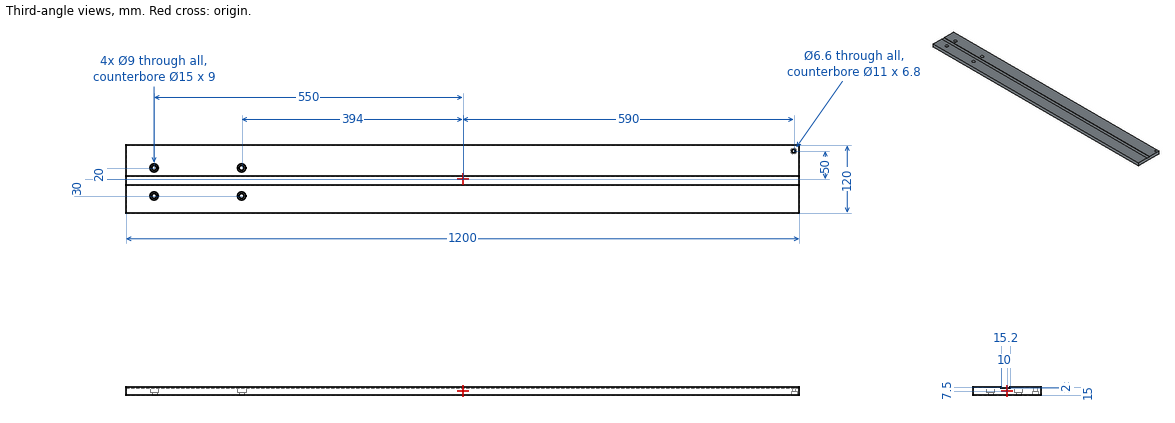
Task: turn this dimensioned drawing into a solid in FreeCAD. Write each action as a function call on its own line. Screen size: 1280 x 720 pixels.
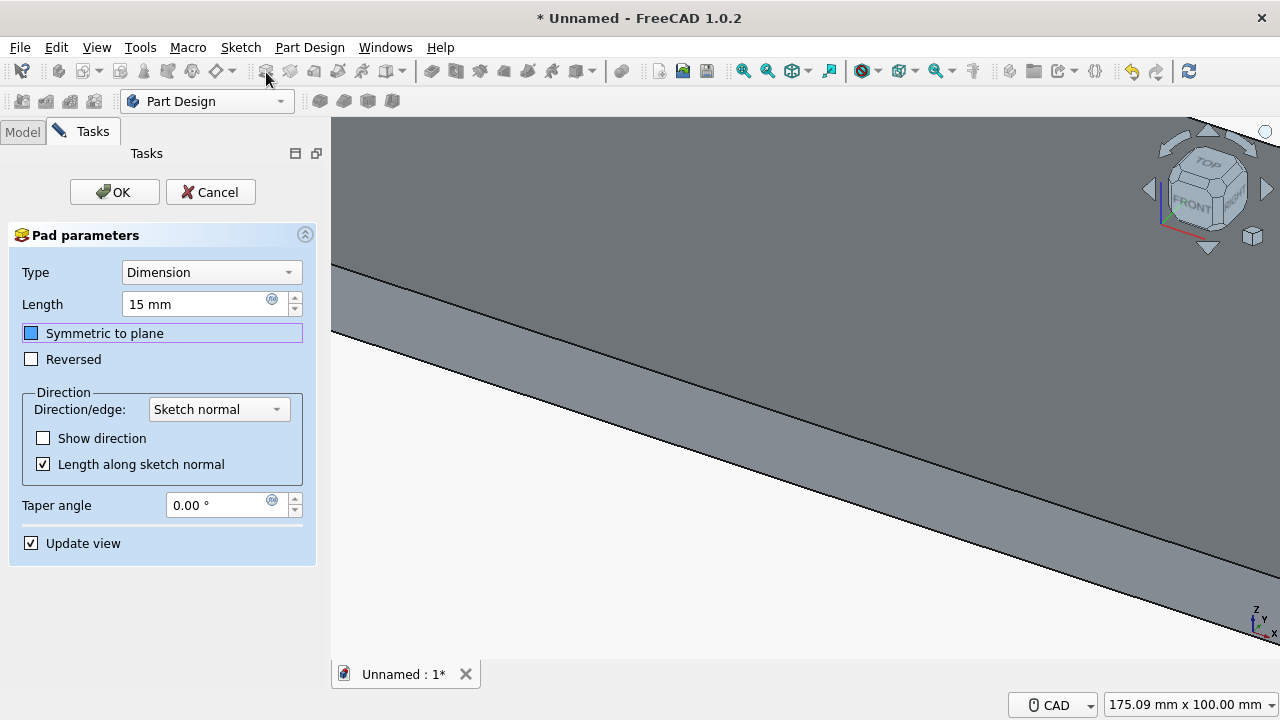
click(30, 333)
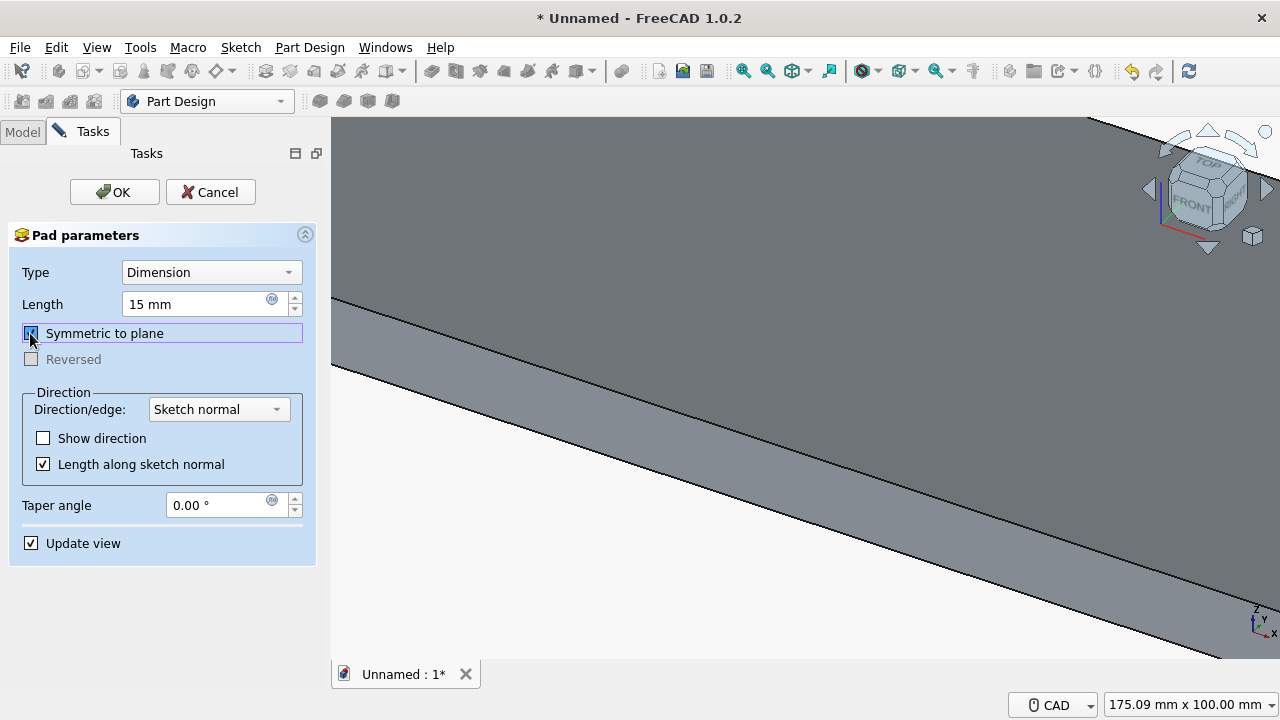
click(115, 192)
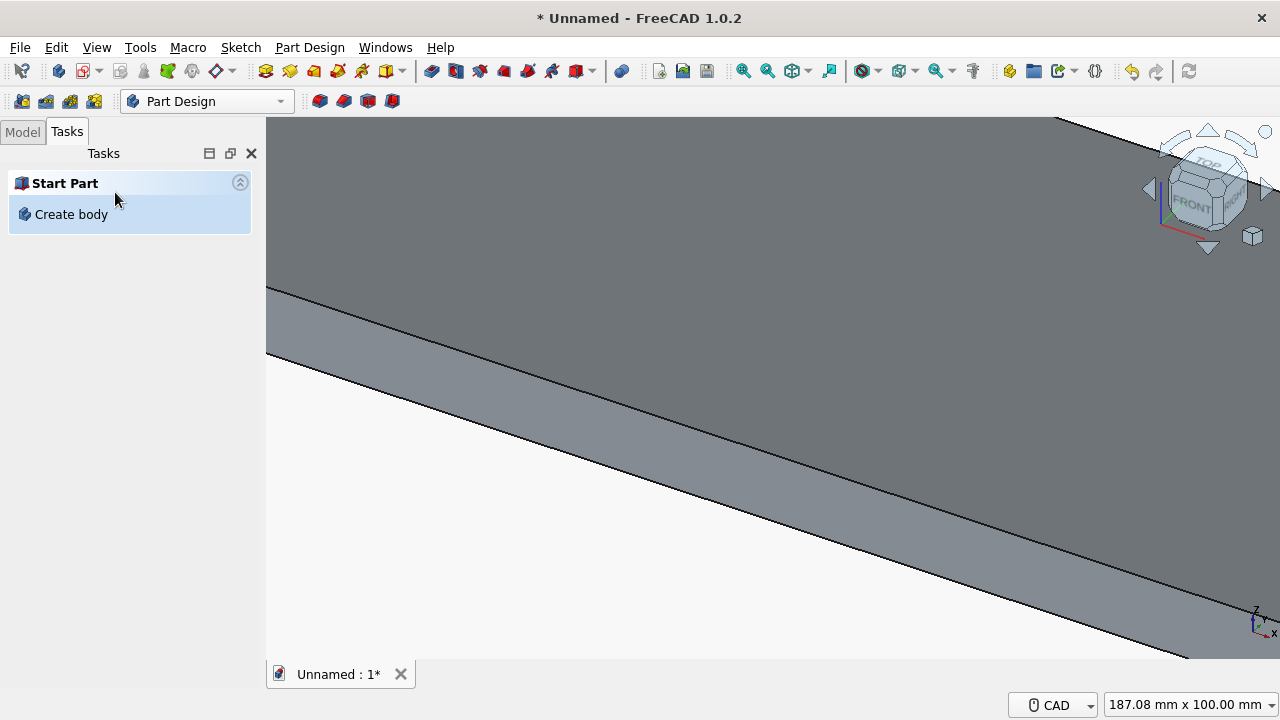
click(744, 72)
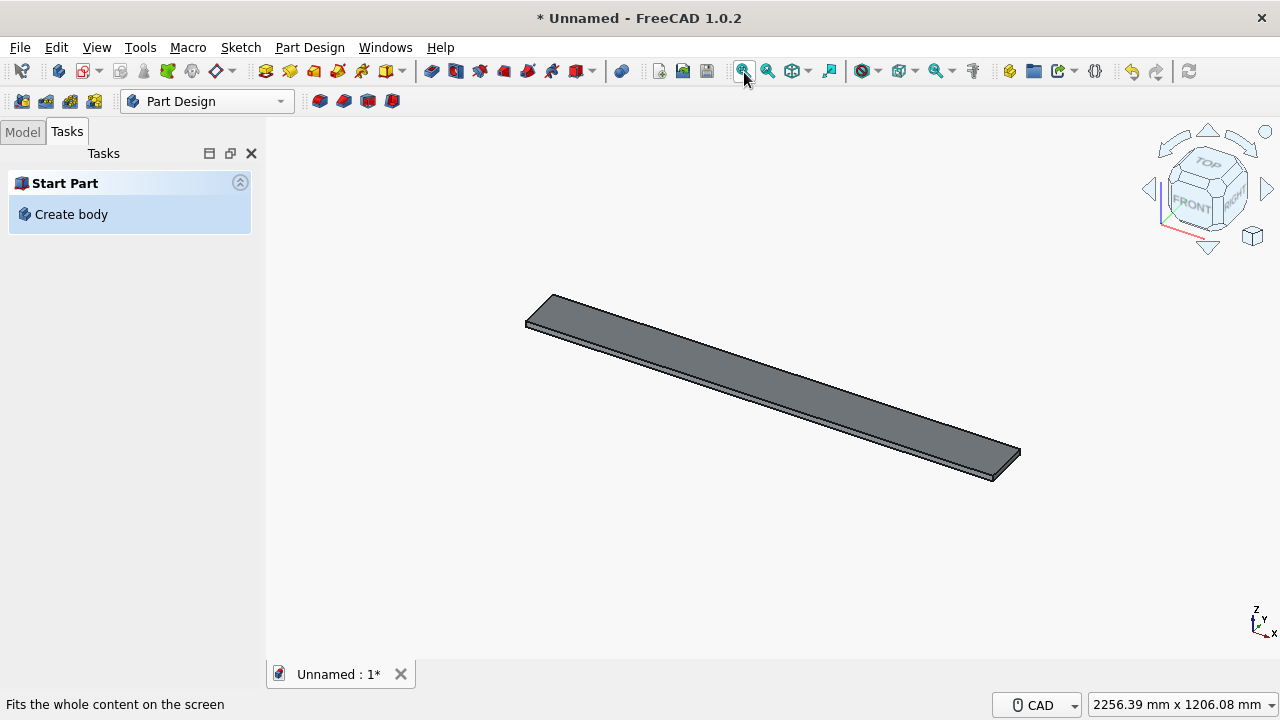
key(5)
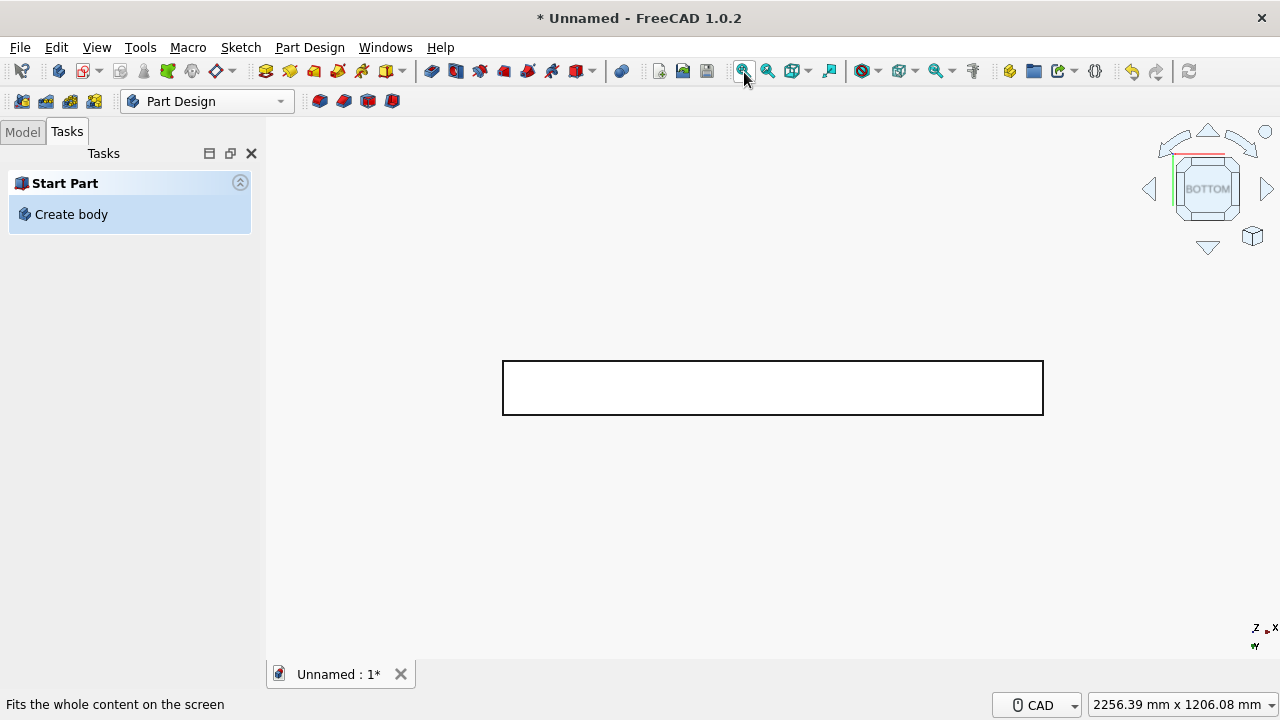
click(1004, 387)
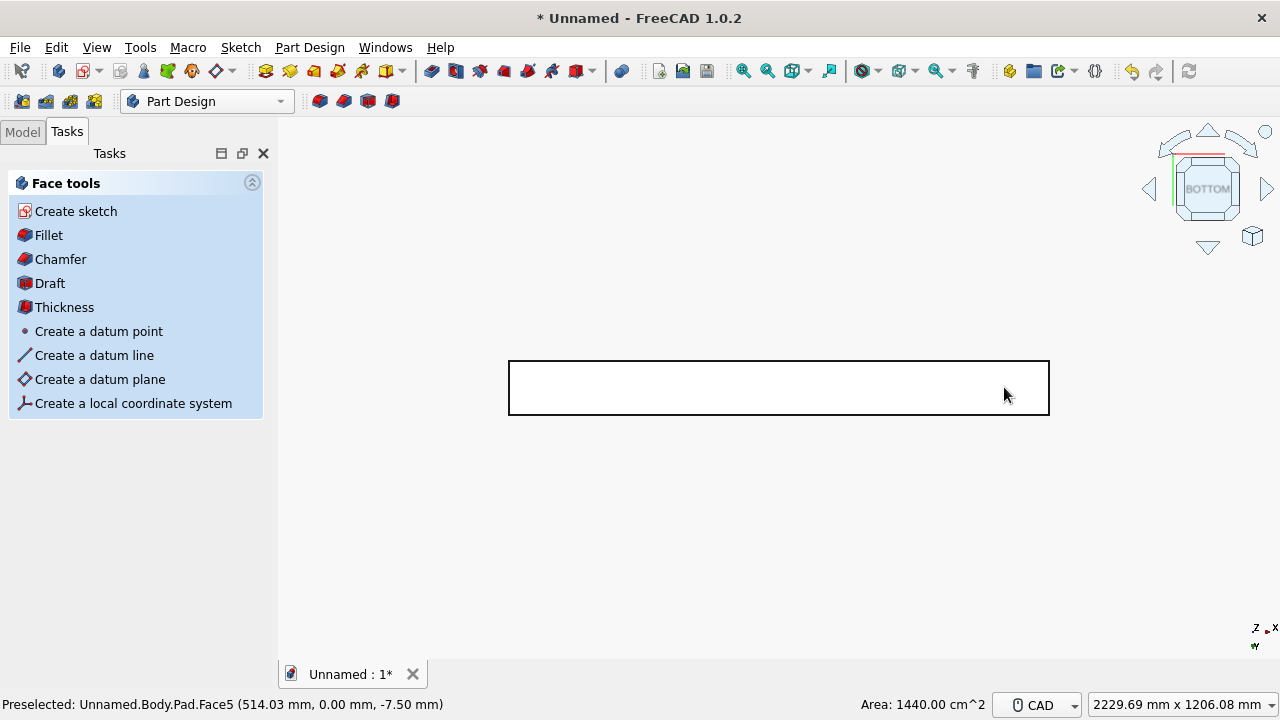
click(84, 72)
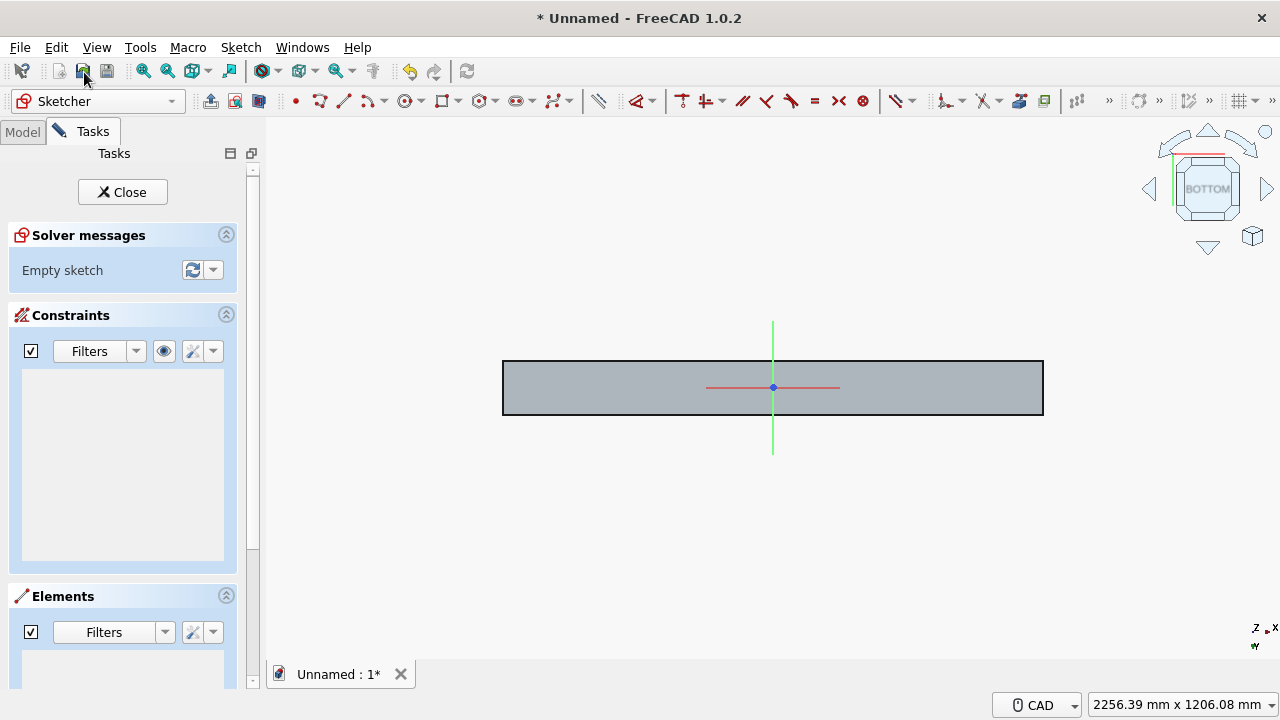
scroll(1056, 412, up, 15)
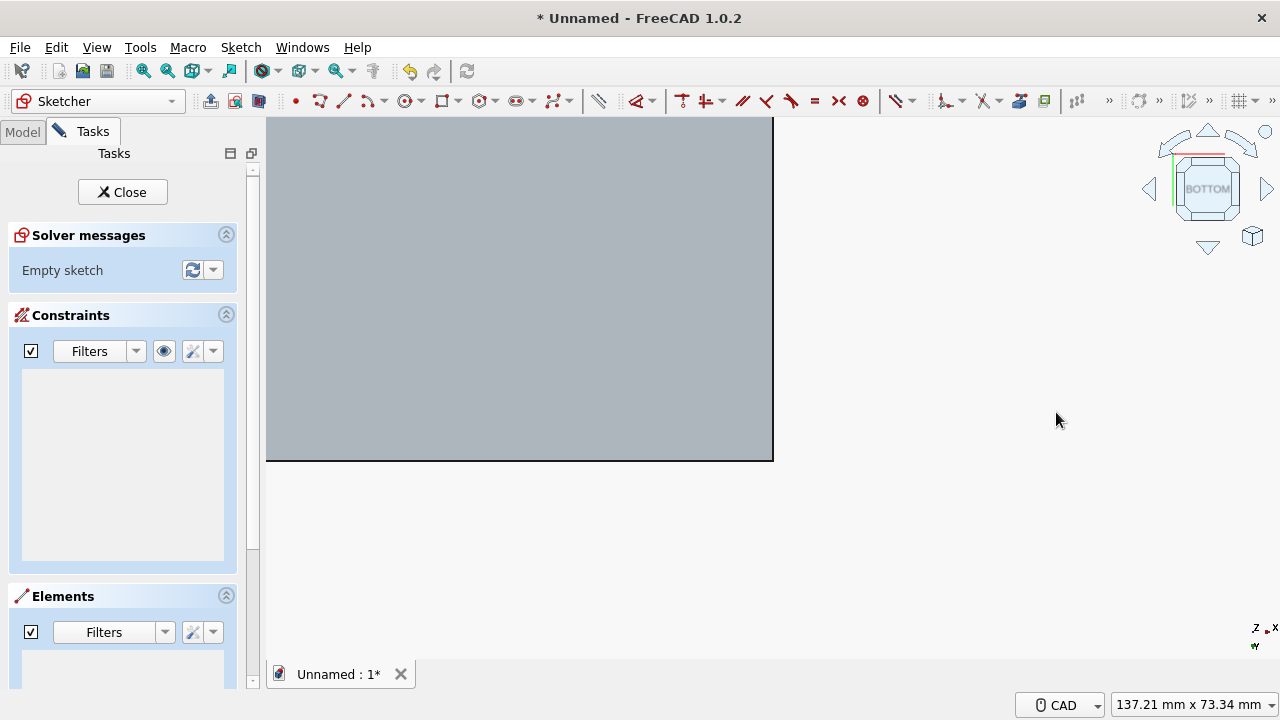
scroll(678, 367, up, 9)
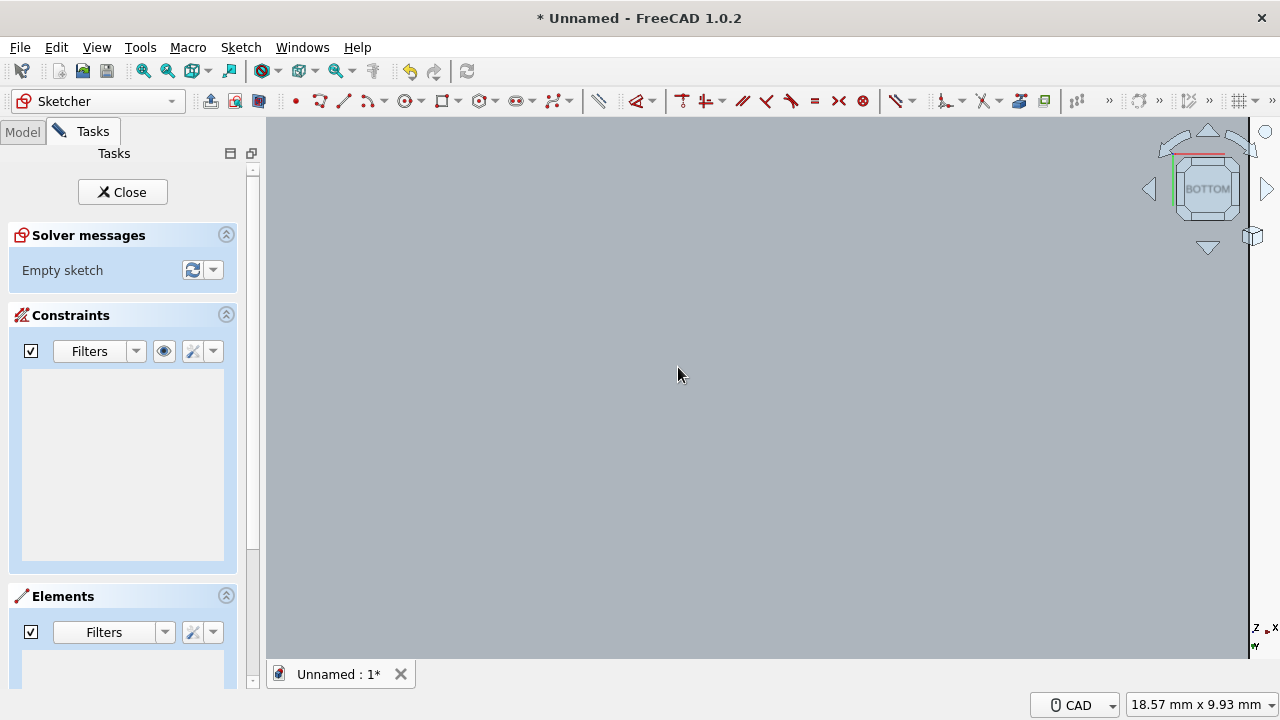
click(406, 102)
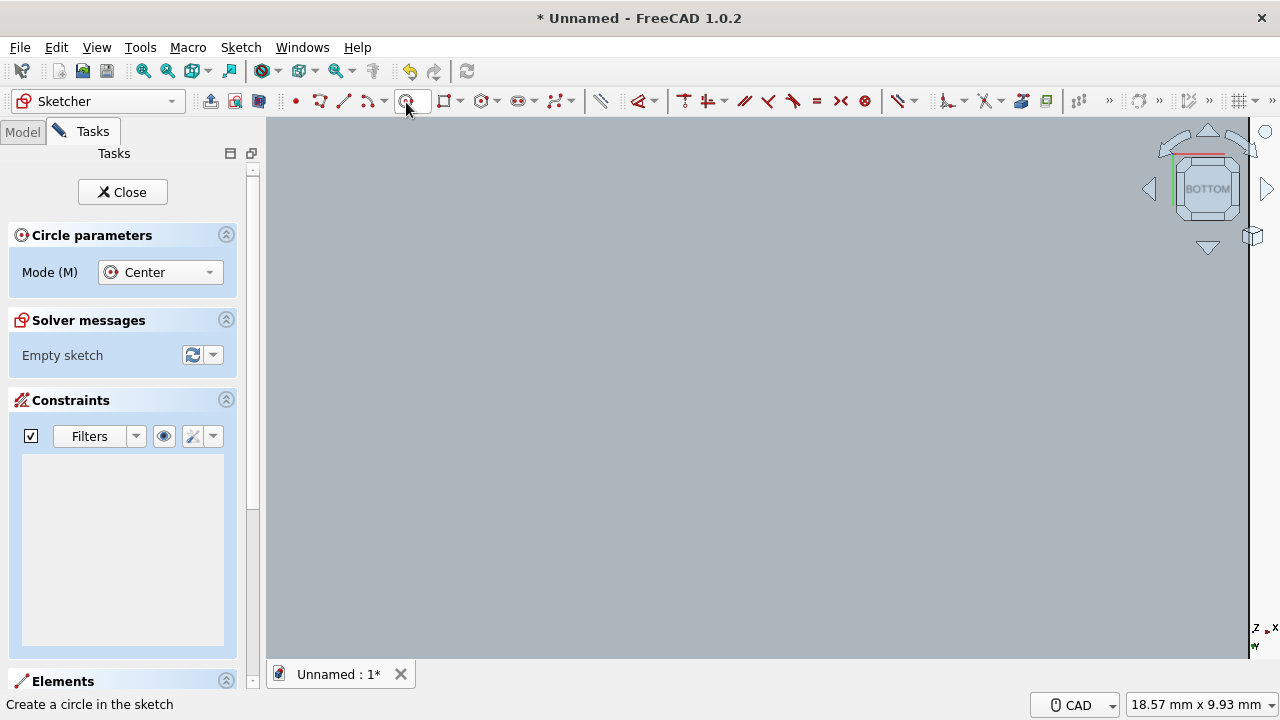
click(703, 388)
move(830, 261)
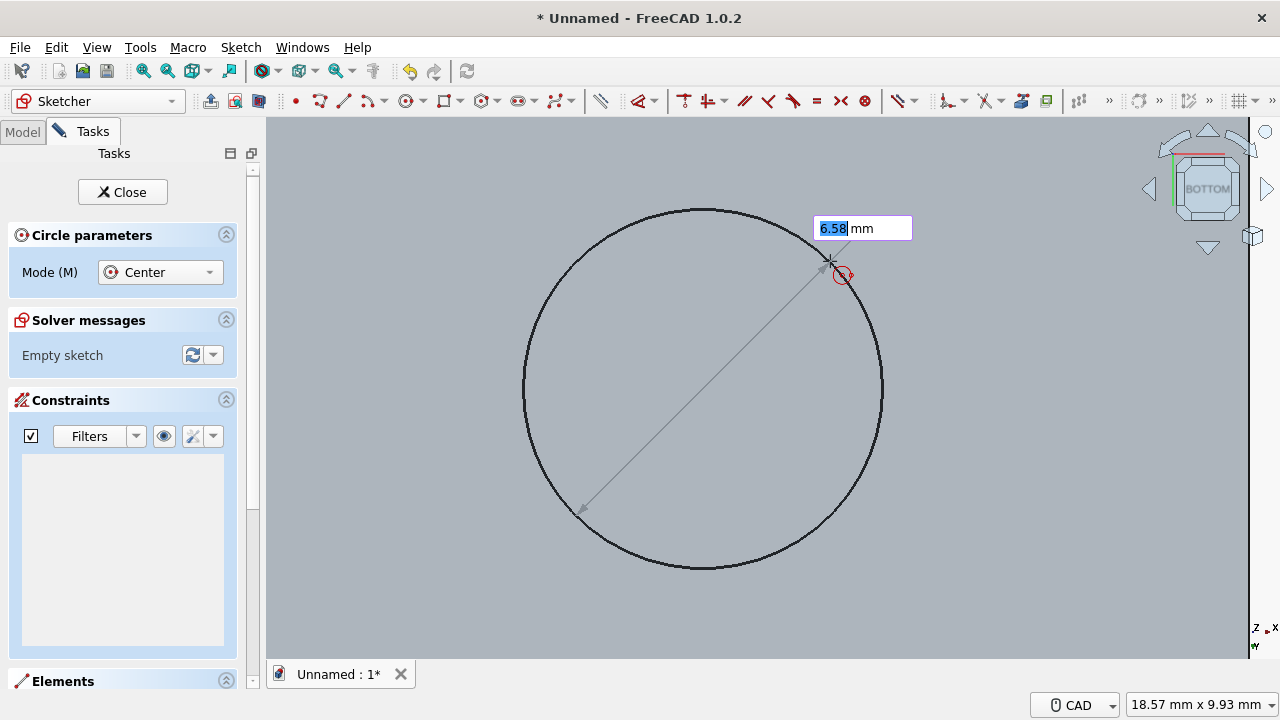
text(6.6)
key(Return)
key(Escape)